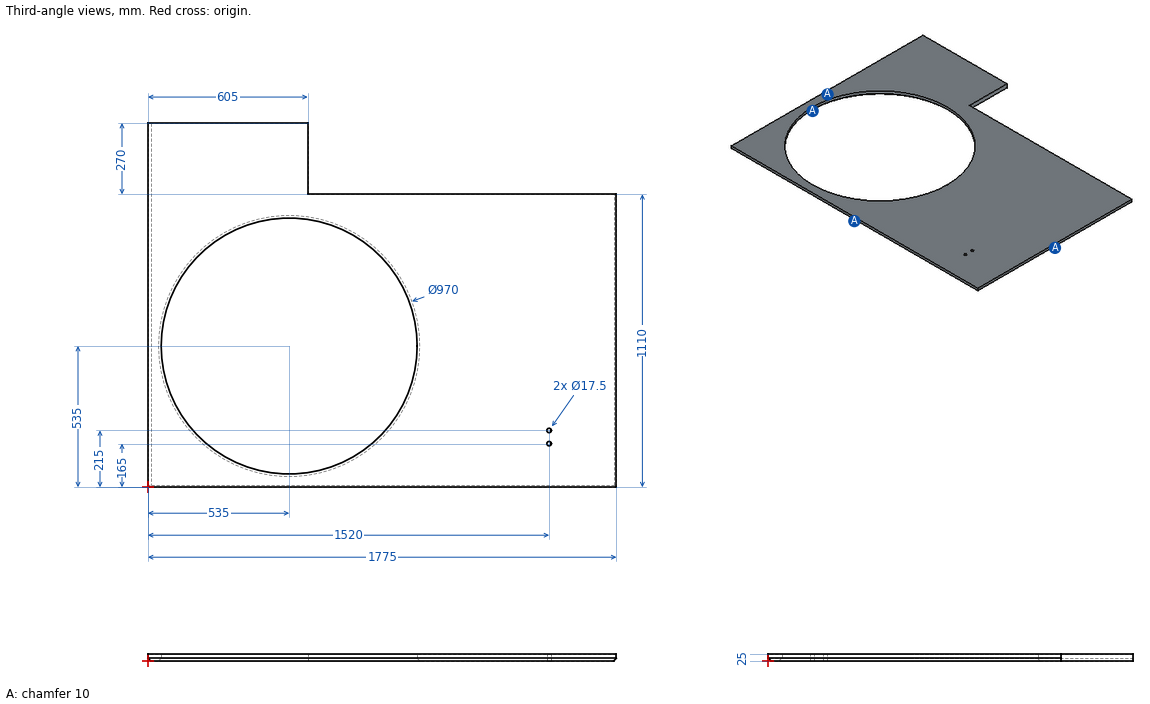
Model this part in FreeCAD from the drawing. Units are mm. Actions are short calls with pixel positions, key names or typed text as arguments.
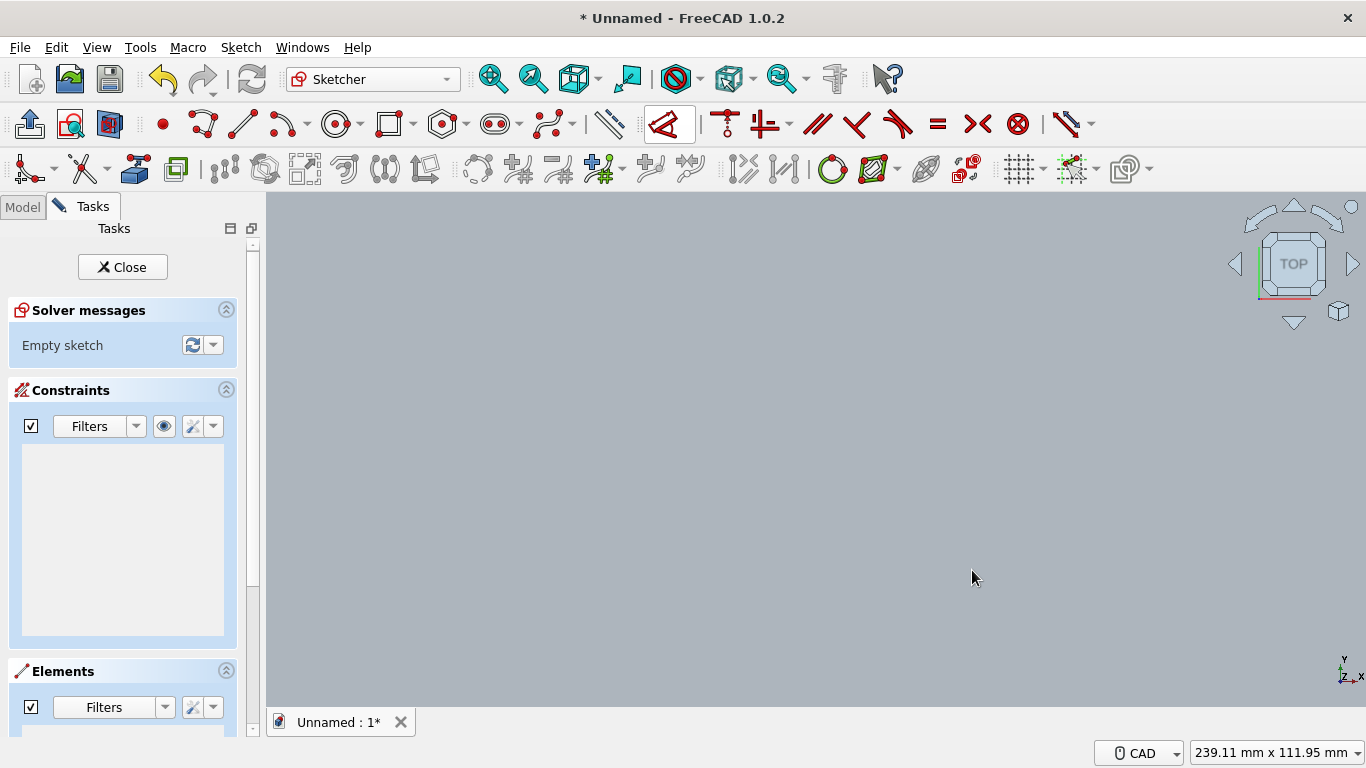
click(336, 124)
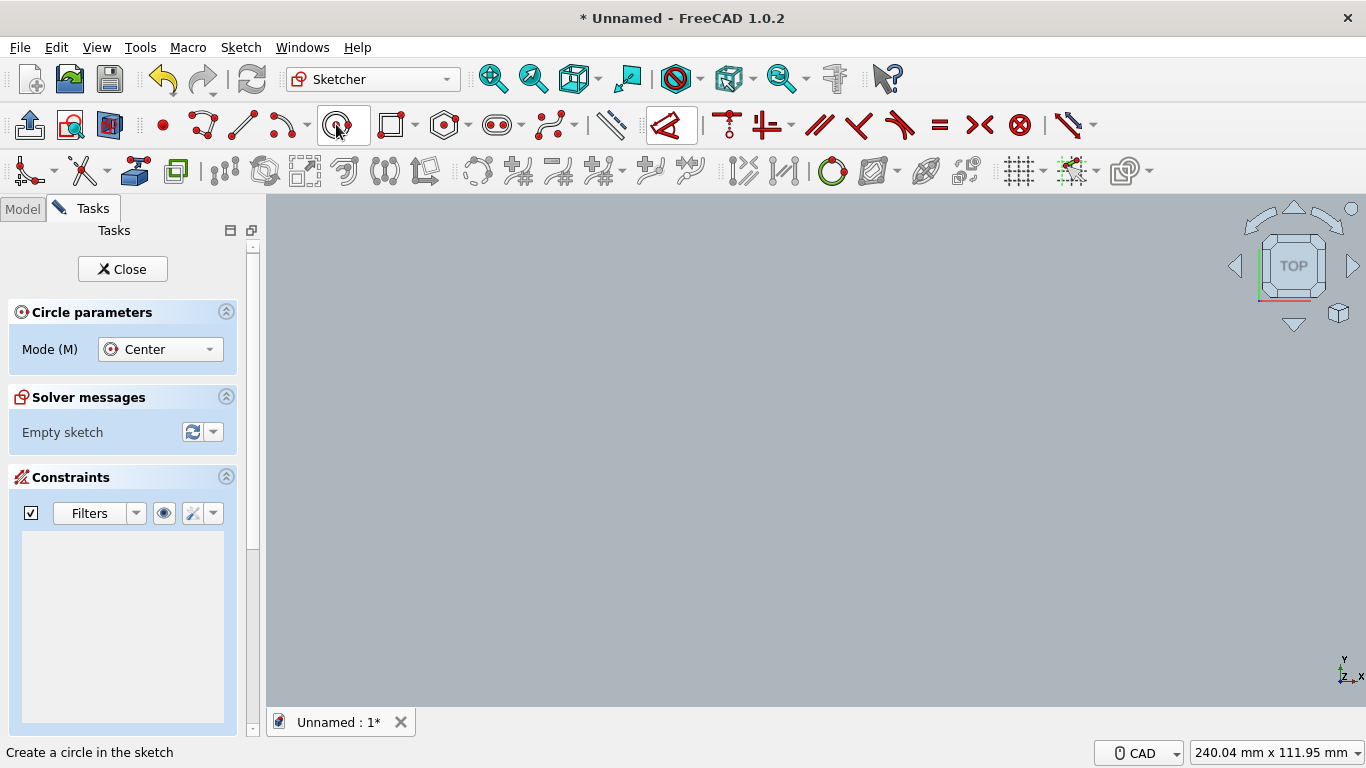
click(737, 322)
click(765, 294)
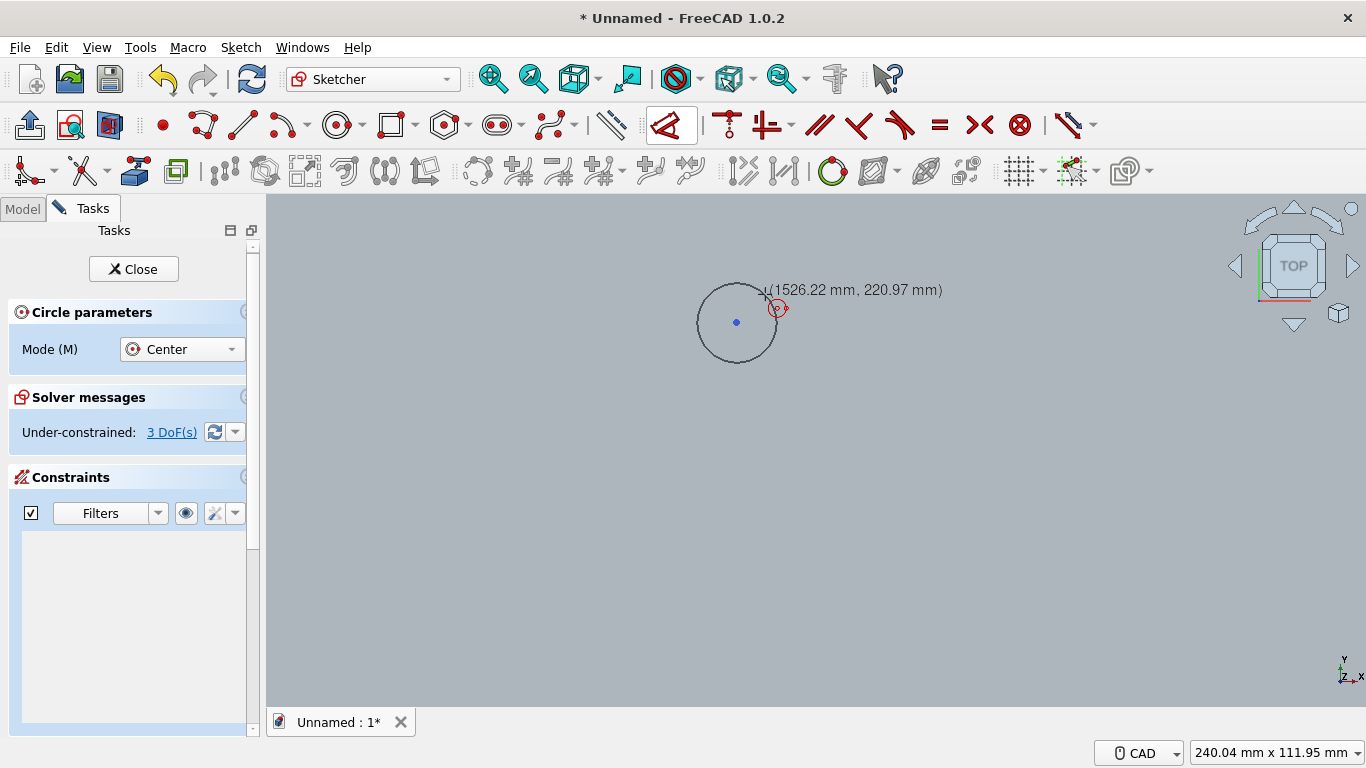
click(737, 552)
click(765, 523)
key(Escape)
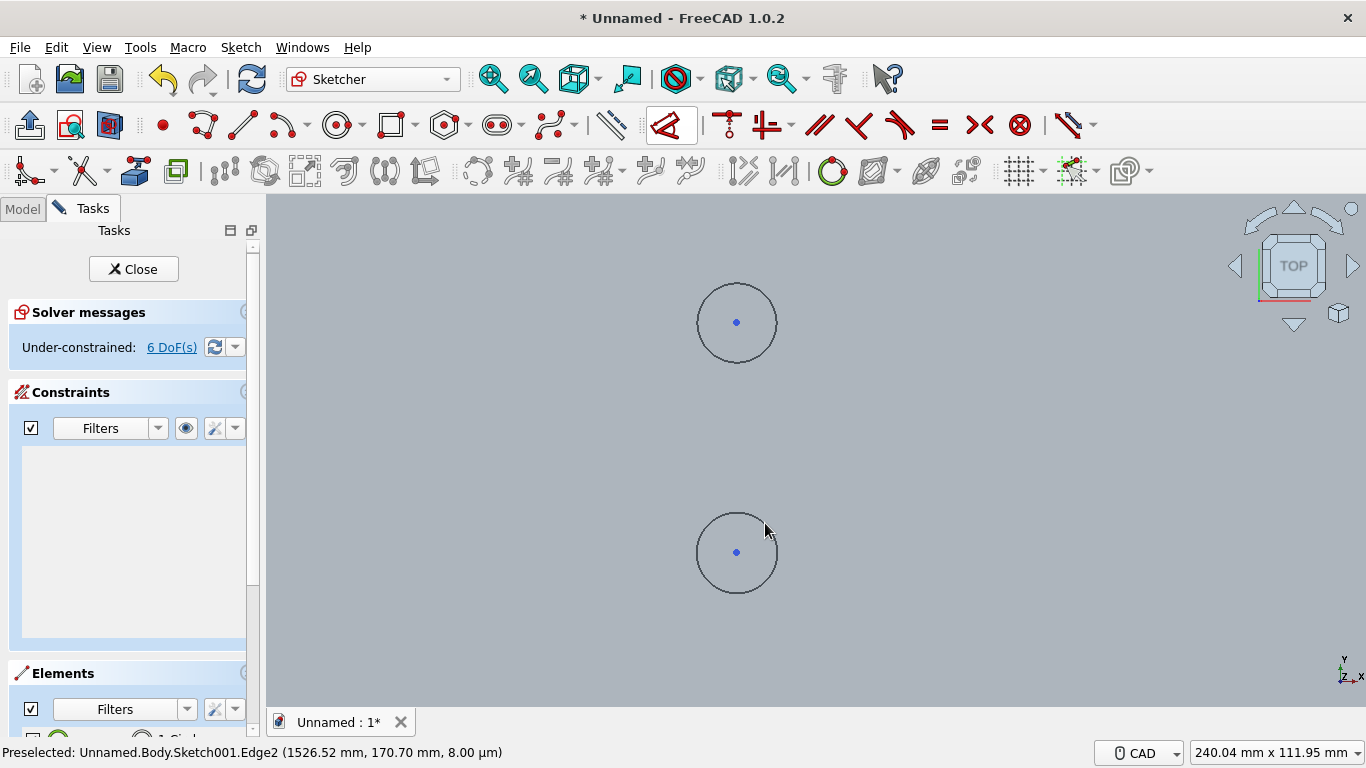
click(765, 295)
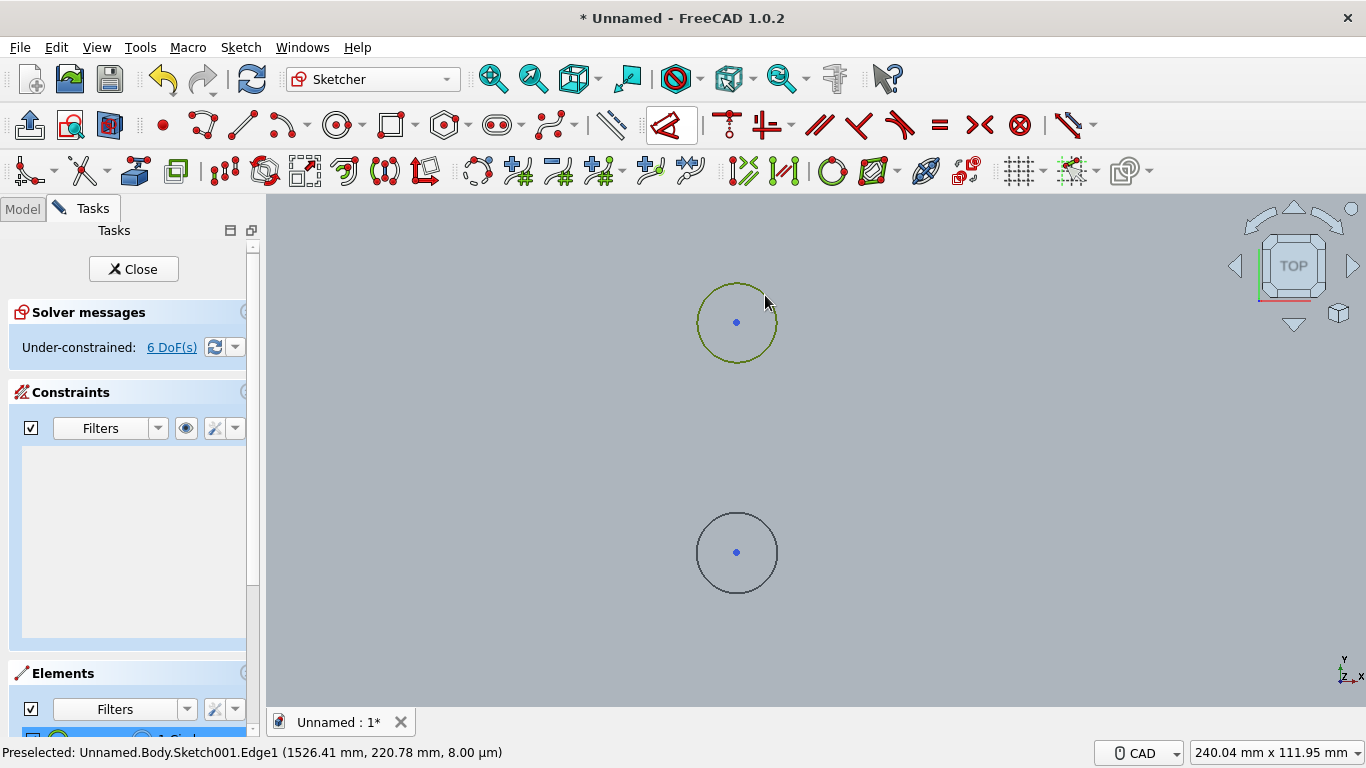
click(765, 524)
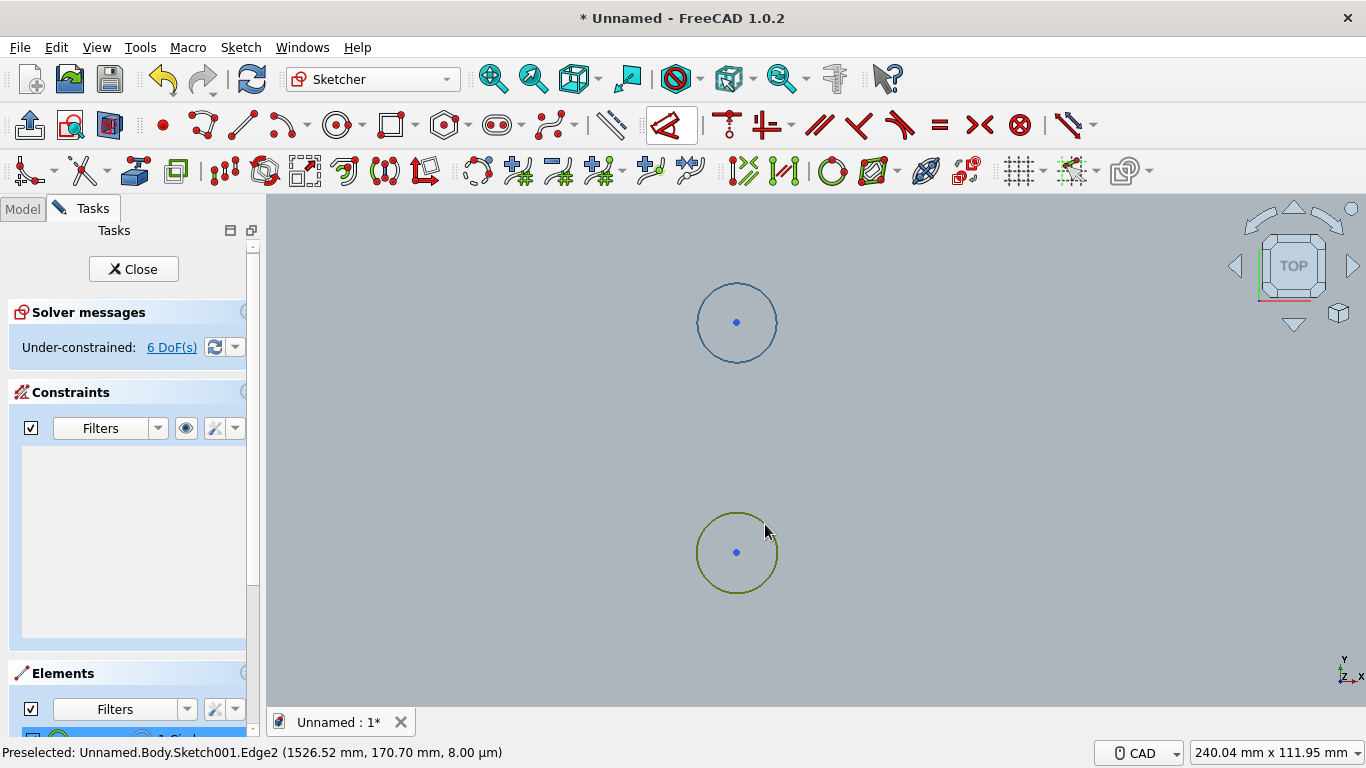
click(940, 126)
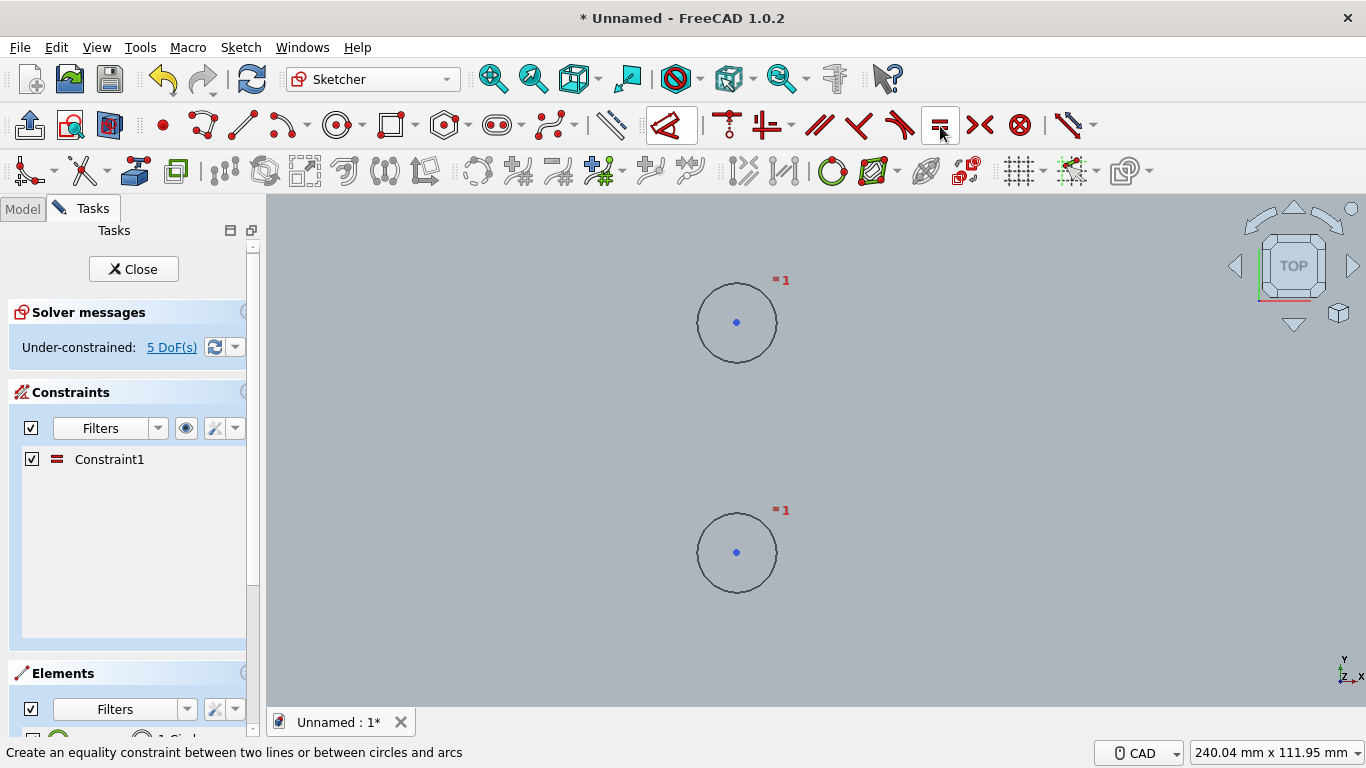
click(737, 323)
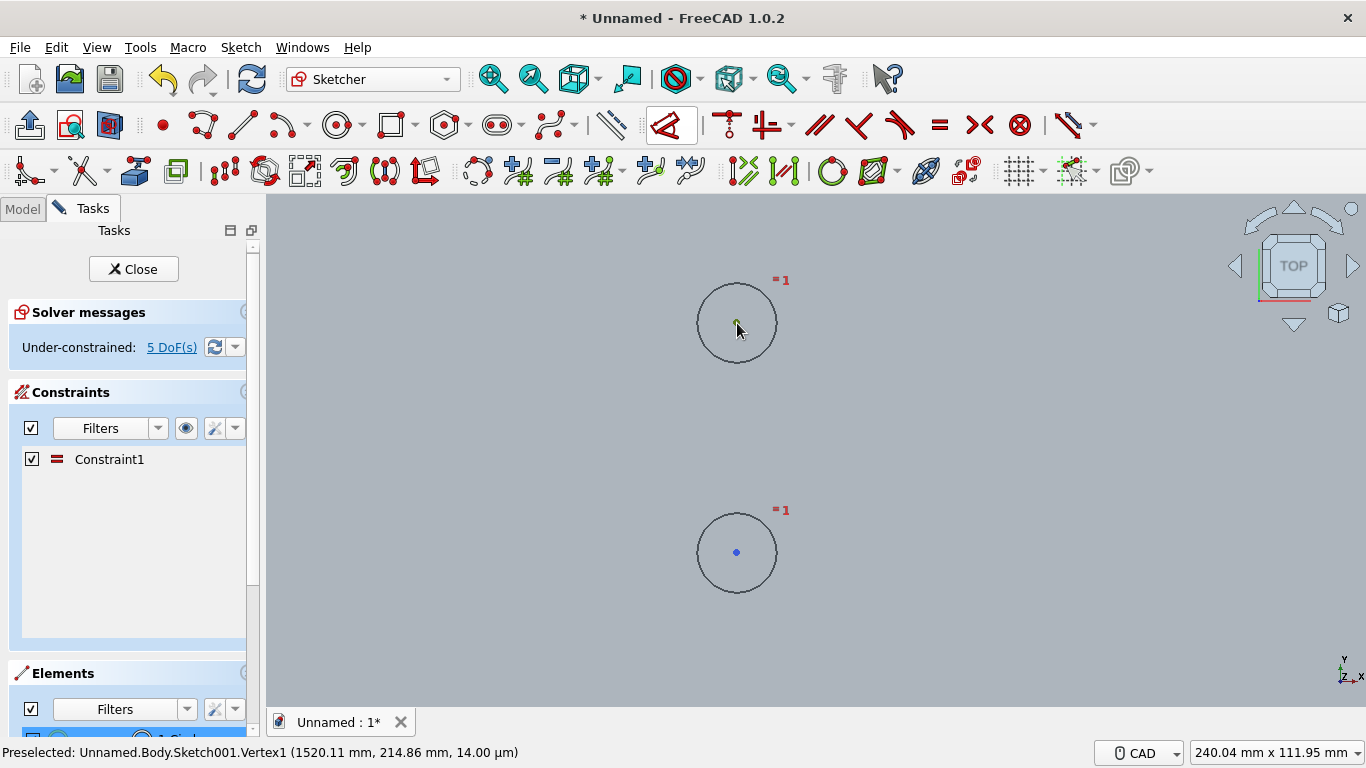
click(737, 553)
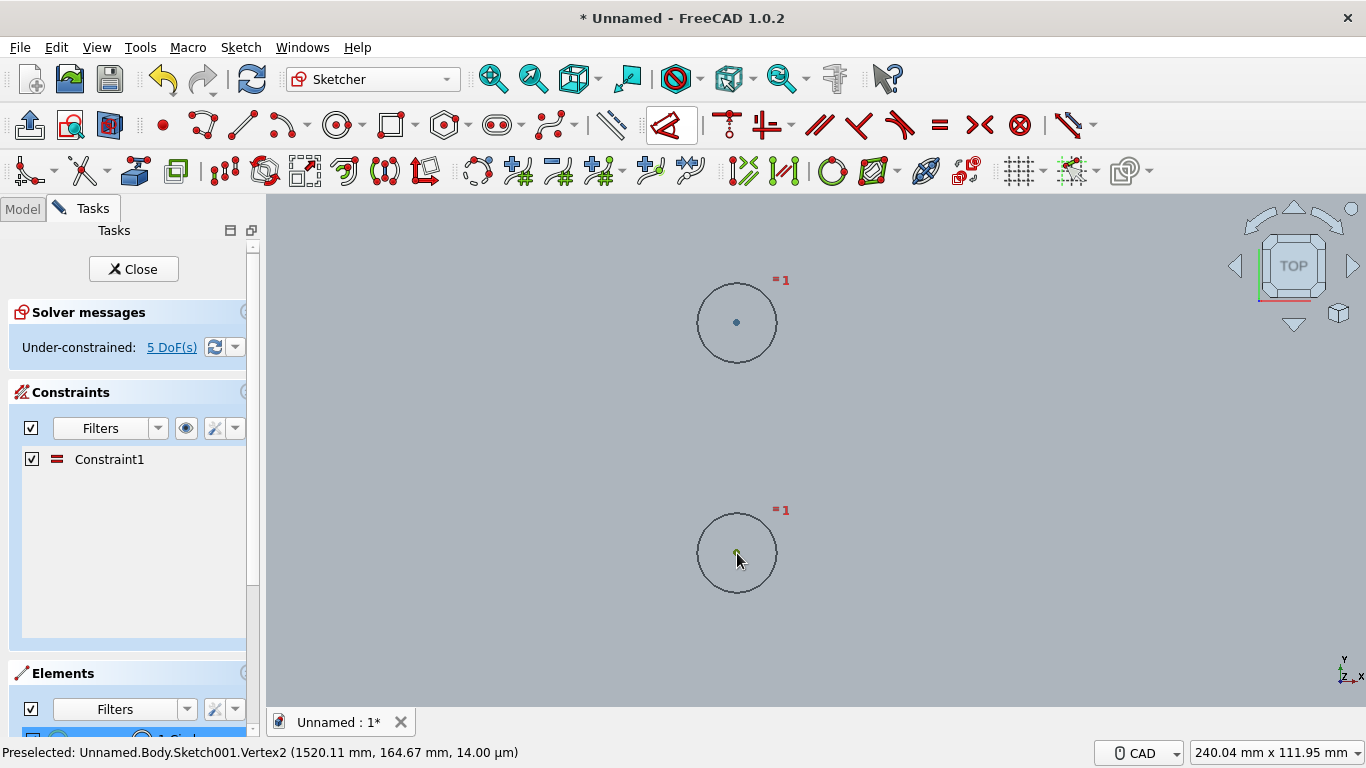
key(v)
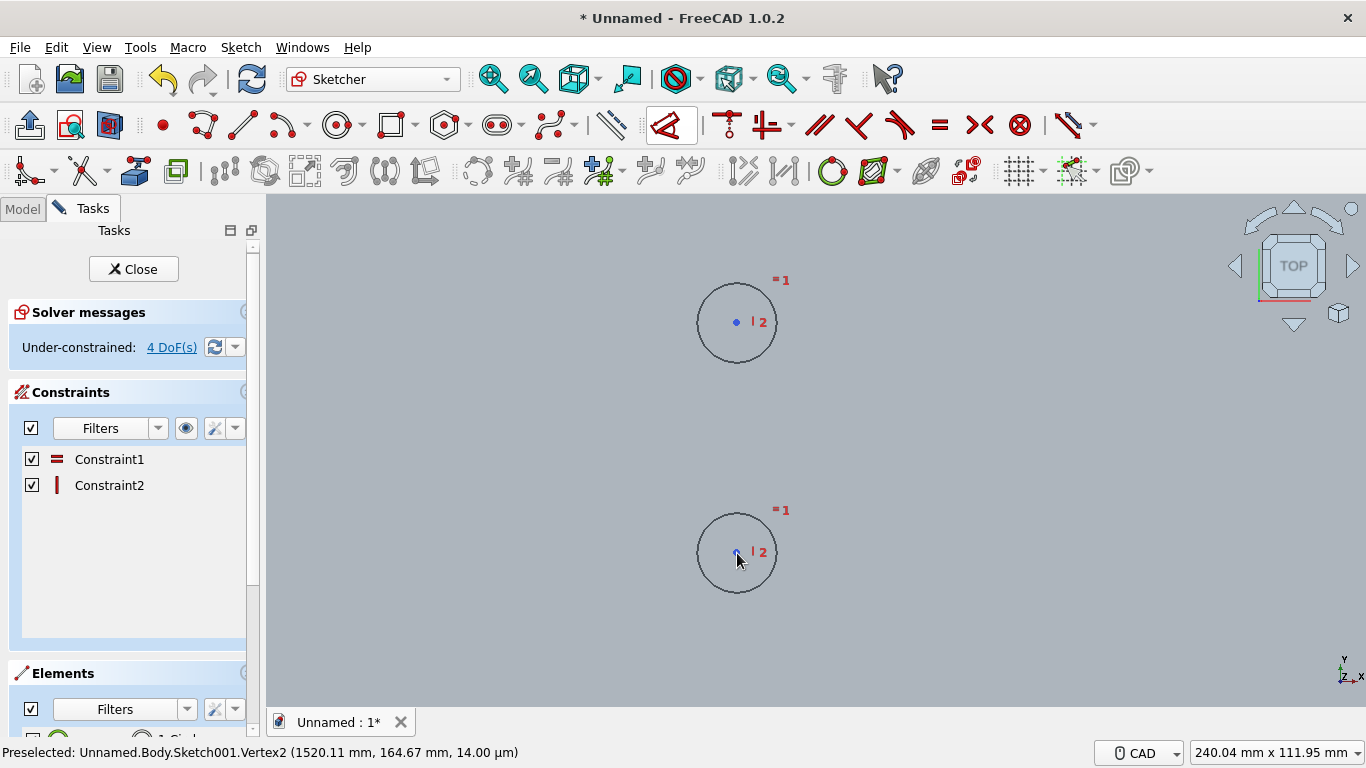
click(765, 295)